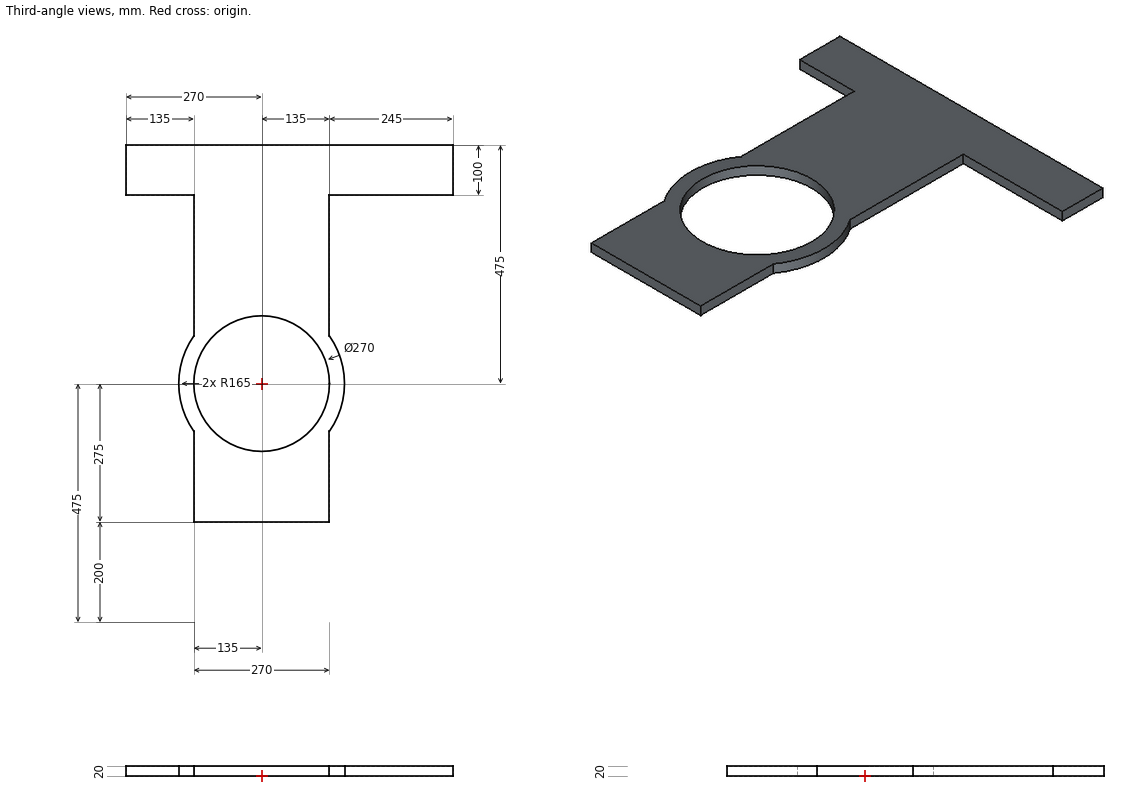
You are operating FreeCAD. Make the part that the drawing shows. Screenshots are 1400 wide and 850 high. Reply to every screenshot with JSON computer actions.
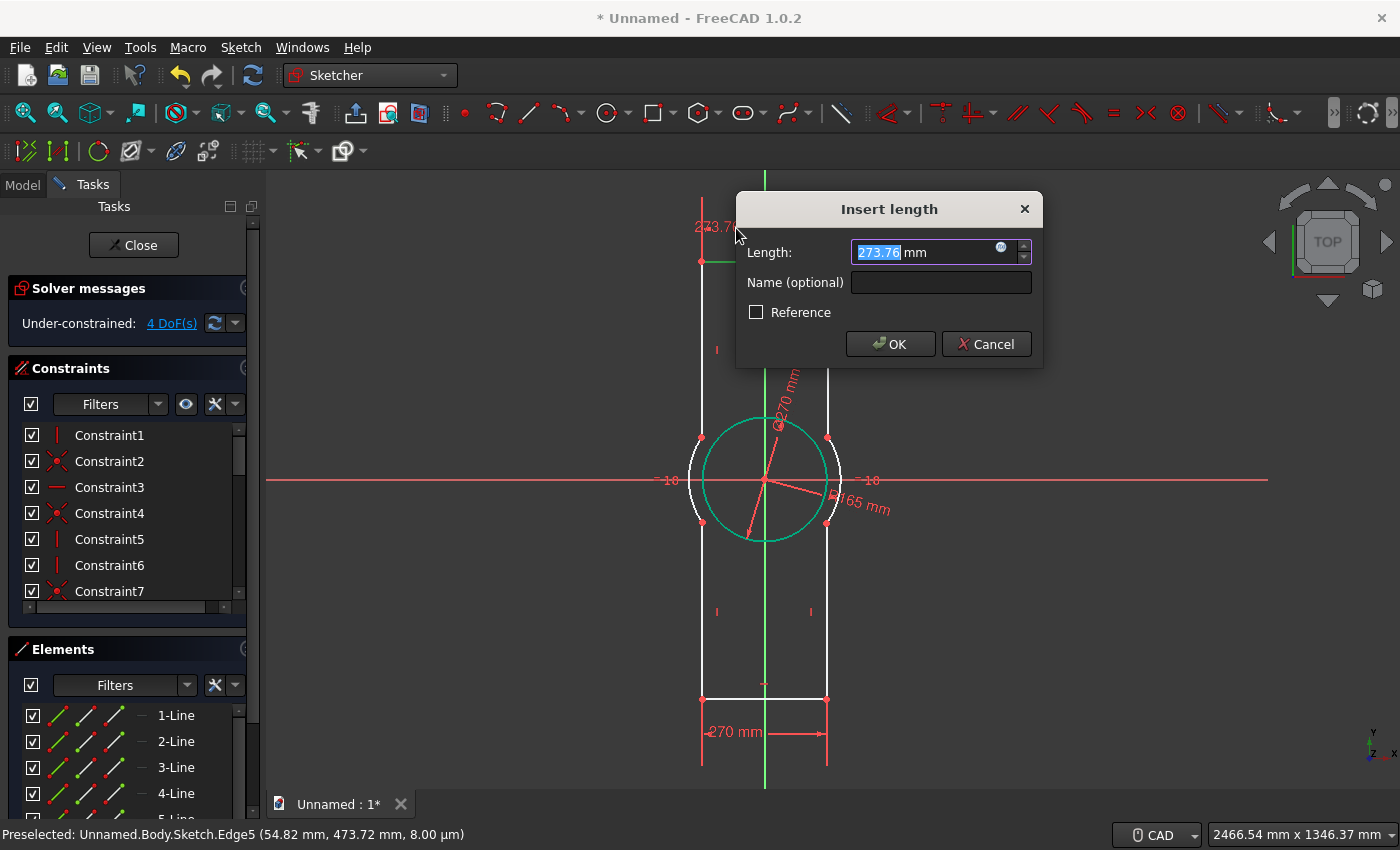
{"action": "type", "text": "270"}
{"action": "key", "text": "Return"}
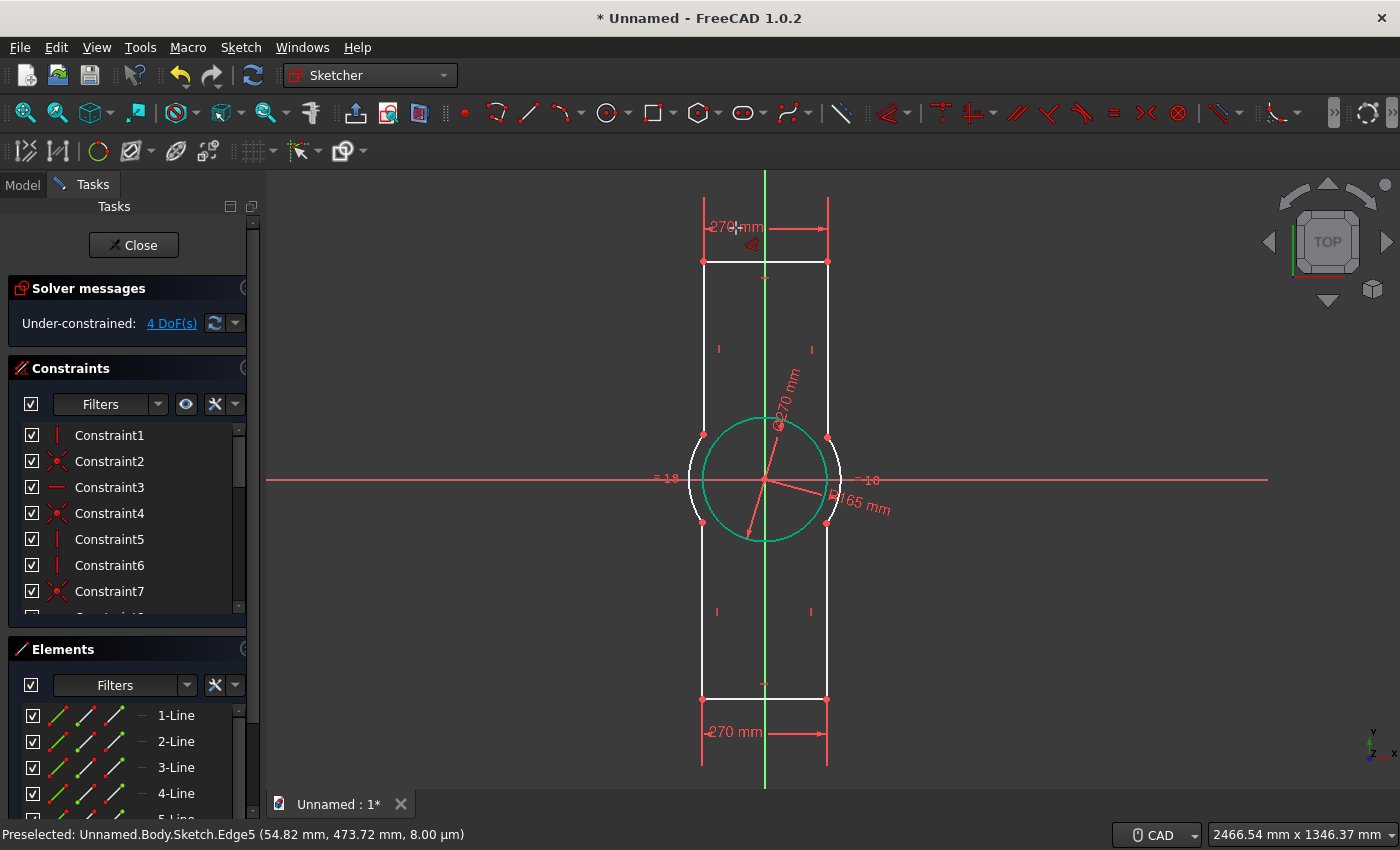
{"action": "left_click", "coordinate": [702, 523]}
{"action": "left_click", "coordinate": [734, 557]}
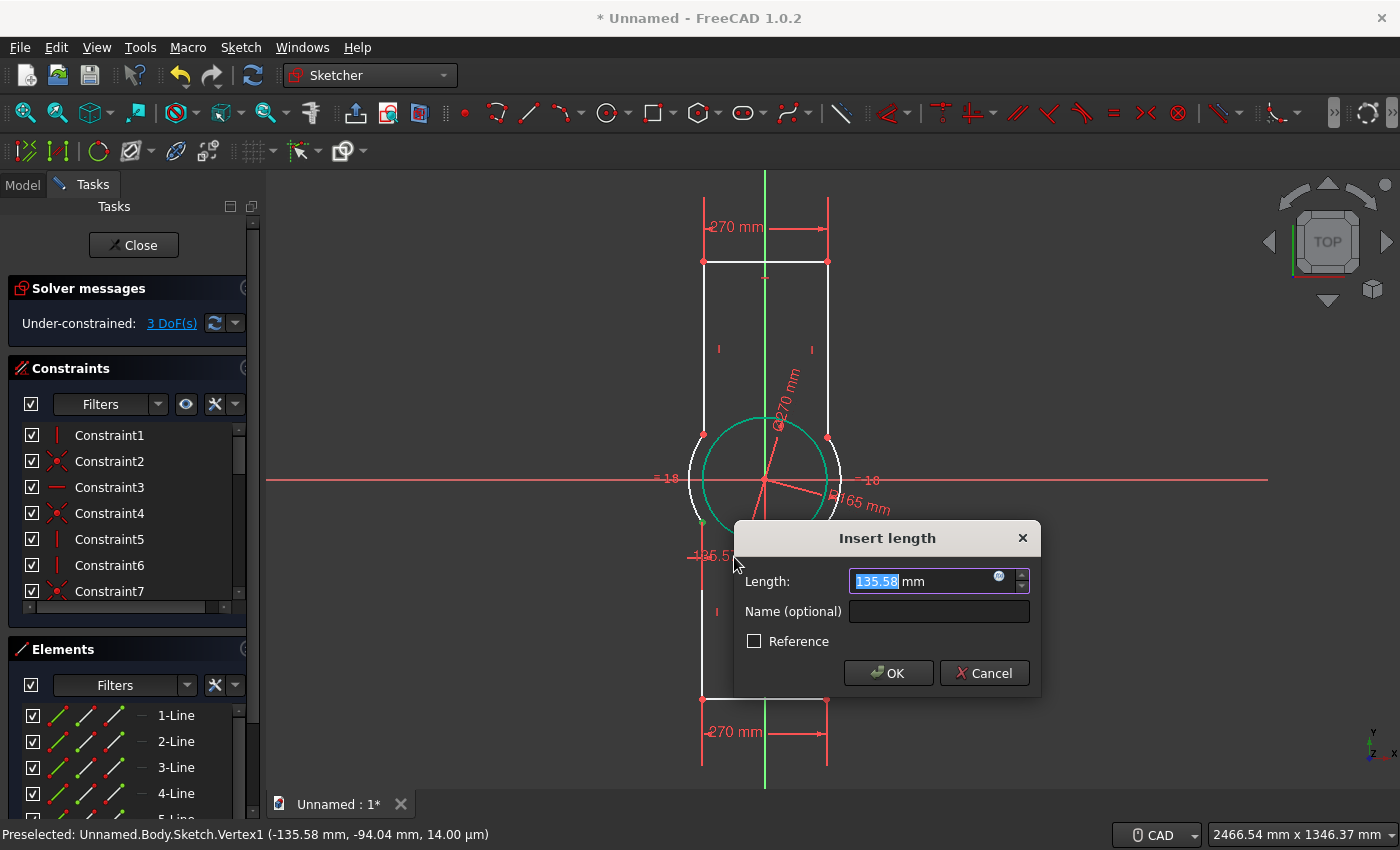
{"action": "type", "text": "135"}
{"action": "key", "text": "Return"}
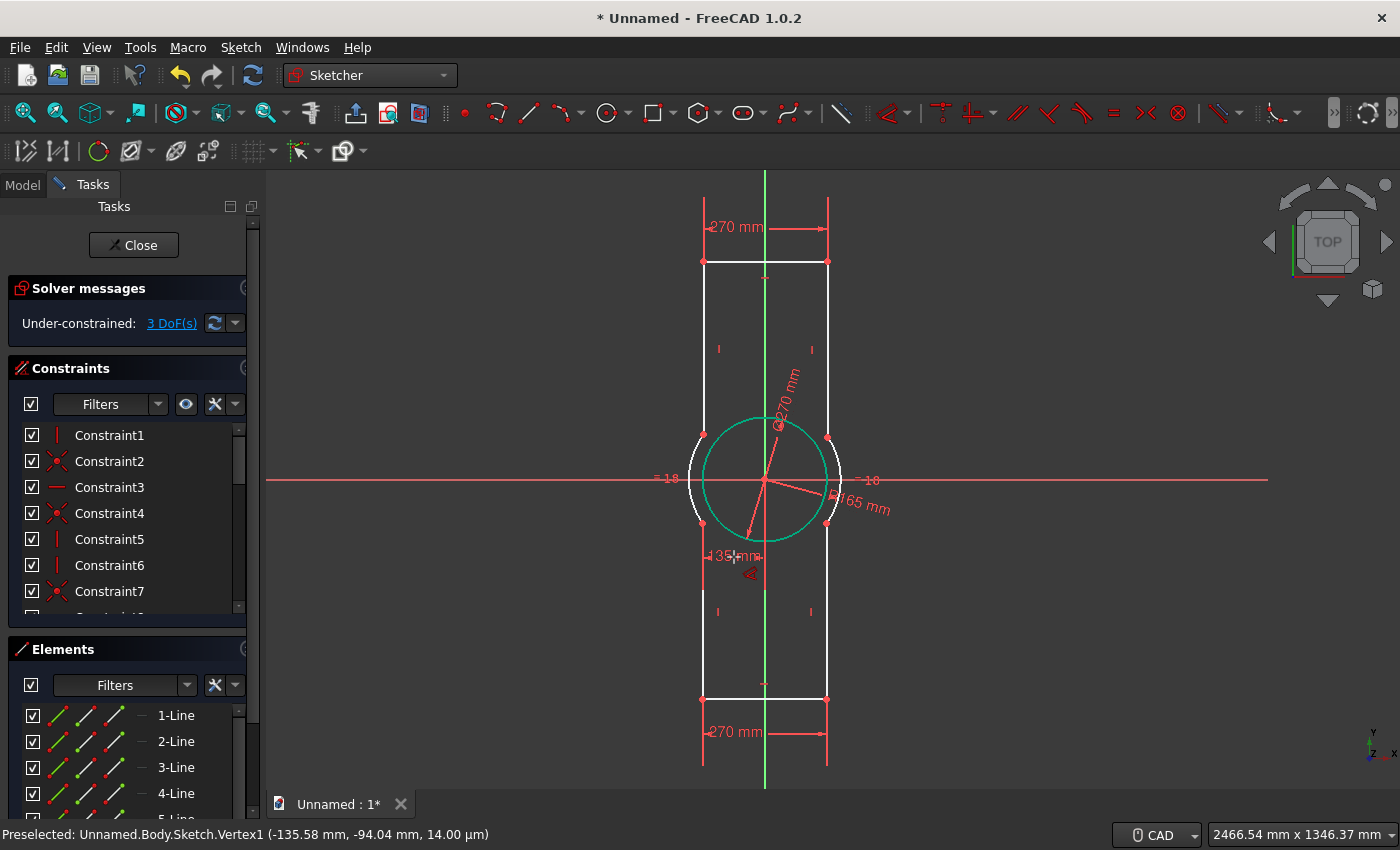
{"action": "left_click", "coordinate": [703, 699]}
{"action": "left_click", "coordinate": [669, 589]}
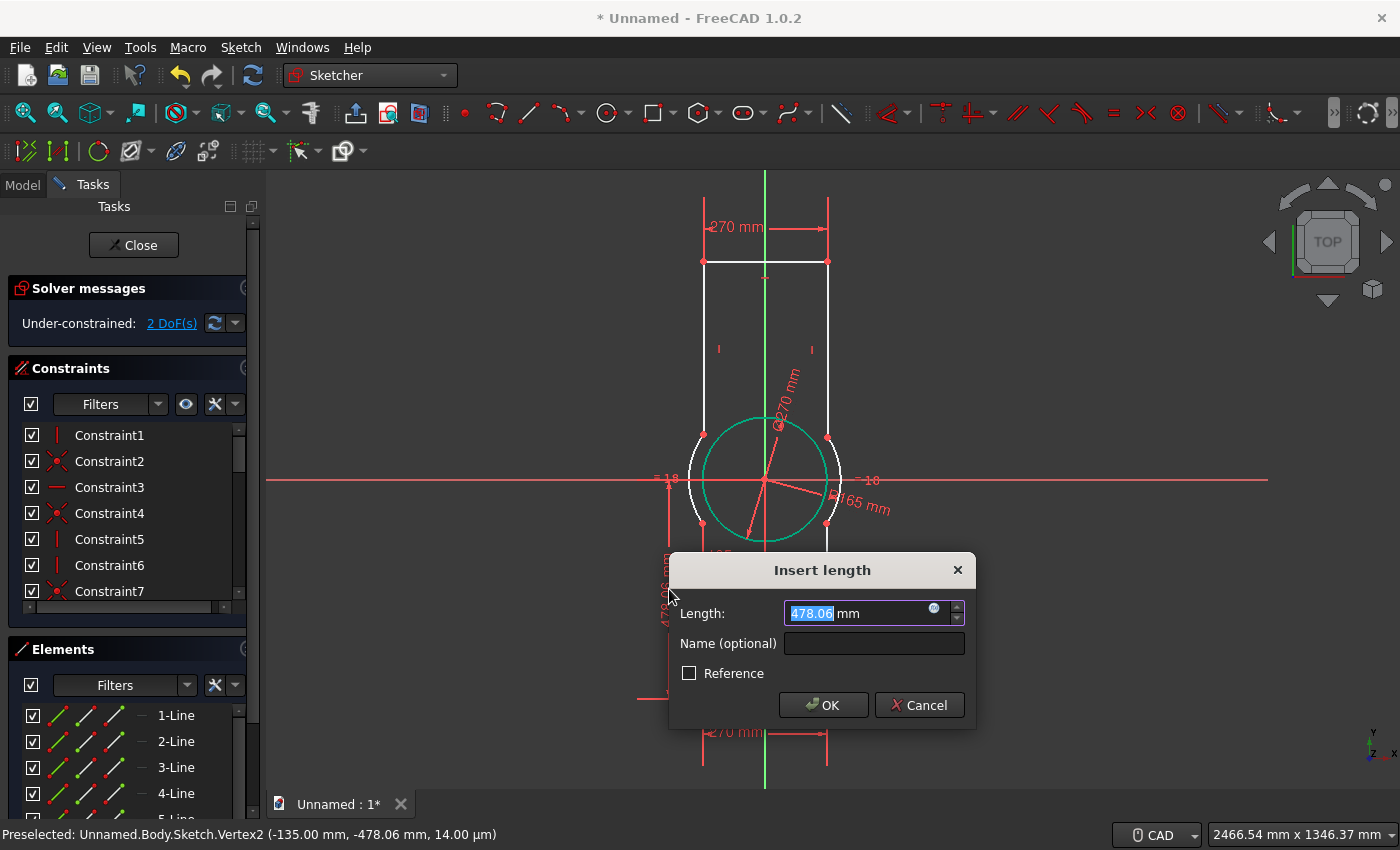
{"action": "type", "text": "475"}
{"action": "key", "text": "Return"}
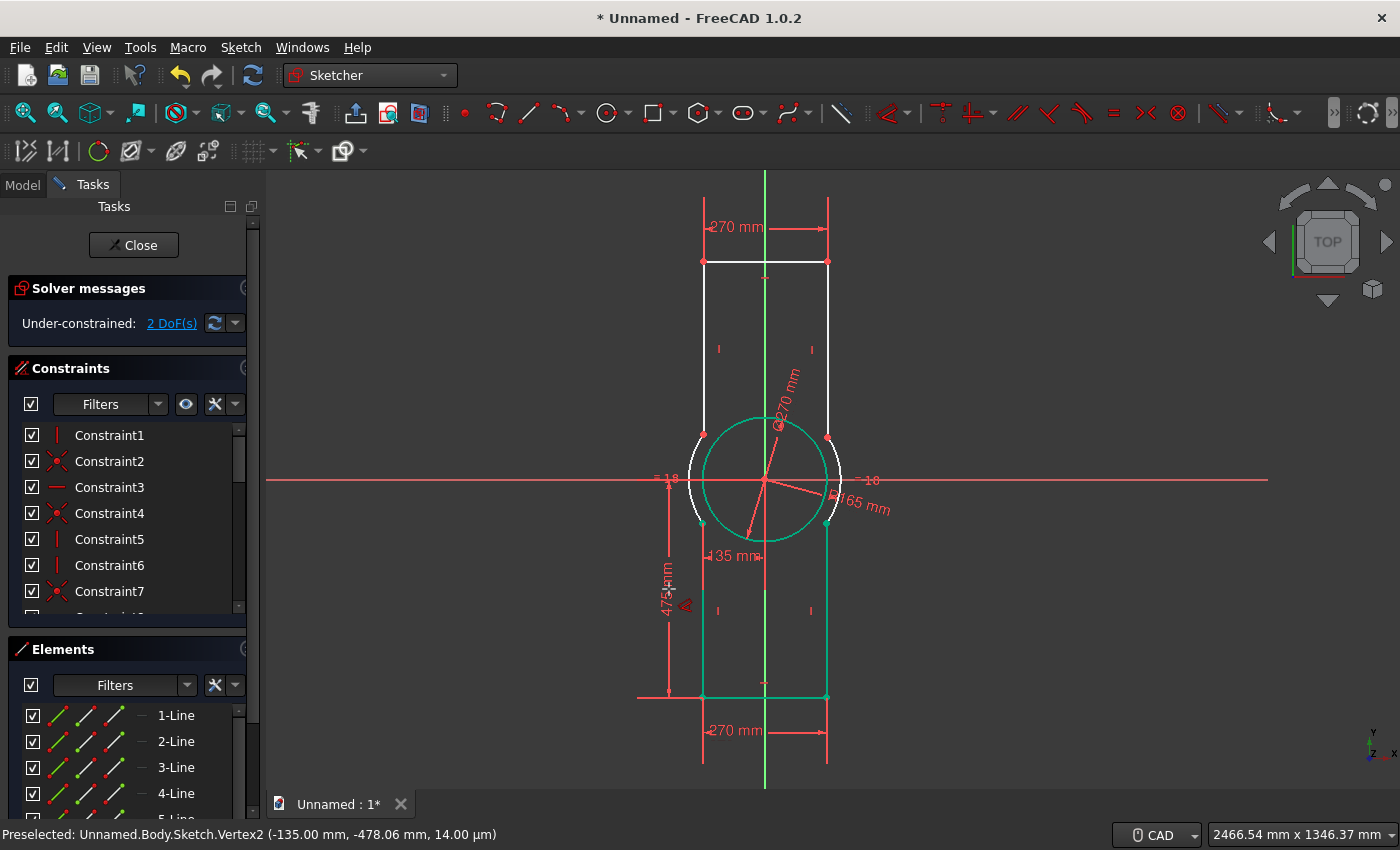
{"action": "left_click", "coordinate": [828, 437]}
{"action": "left_click", "coordinate": [782, 514]}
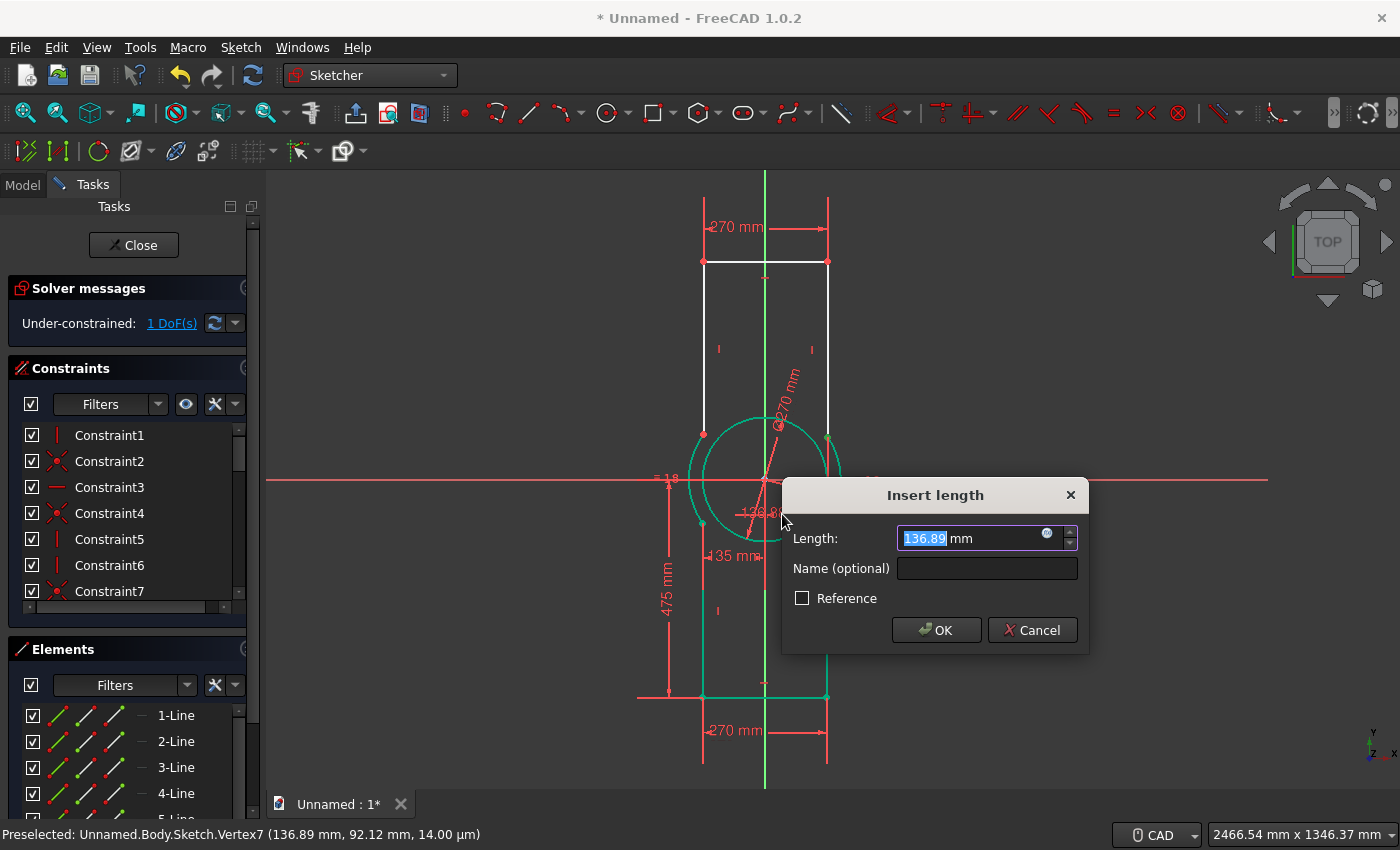
{"action": "type", "text": "135"}
{"action": "key", "text": "Return"}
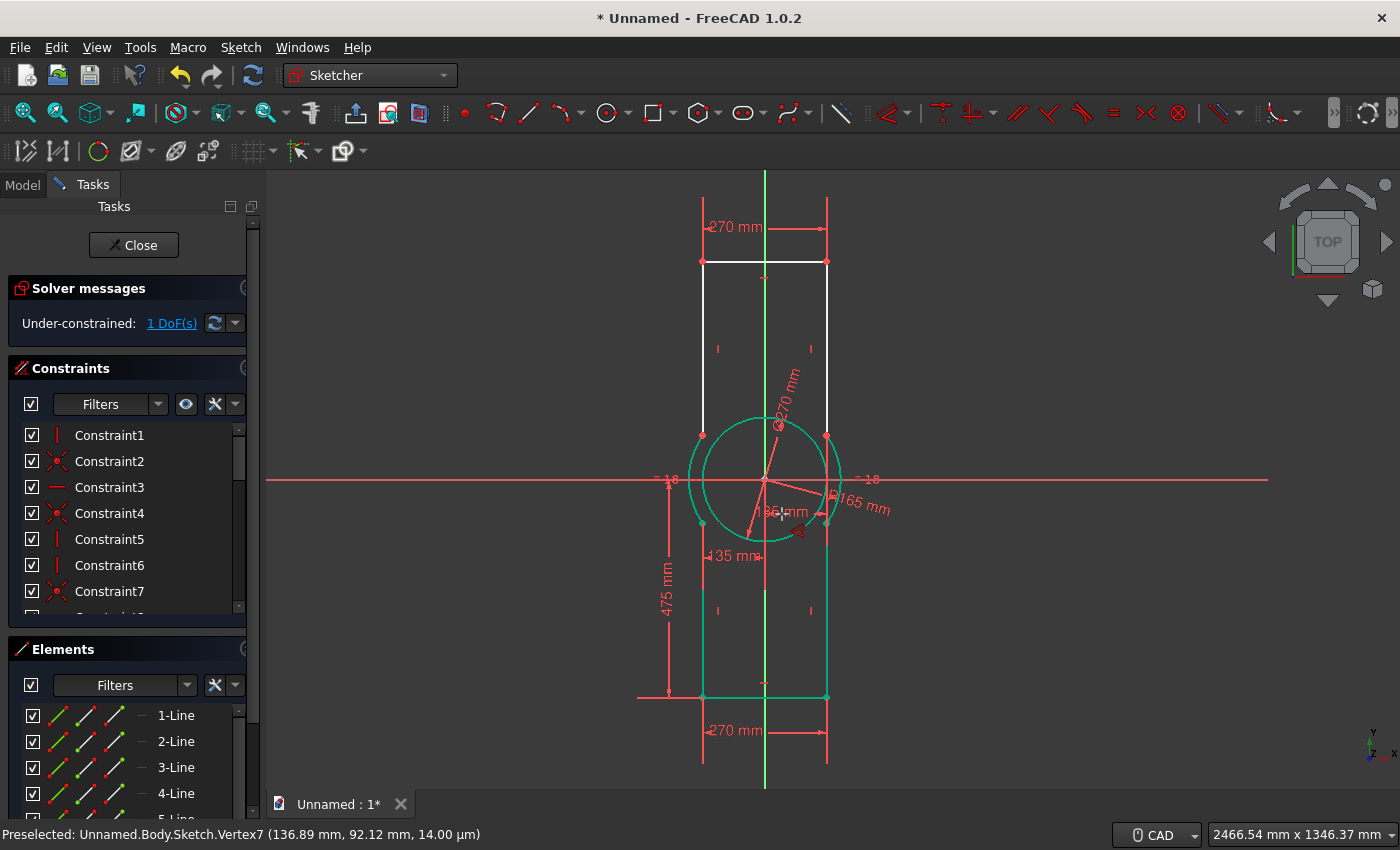
{"action": "left_click", "coordinate": [827, 262]}
{"action": "left_click", "coordinate": [861, 371]}